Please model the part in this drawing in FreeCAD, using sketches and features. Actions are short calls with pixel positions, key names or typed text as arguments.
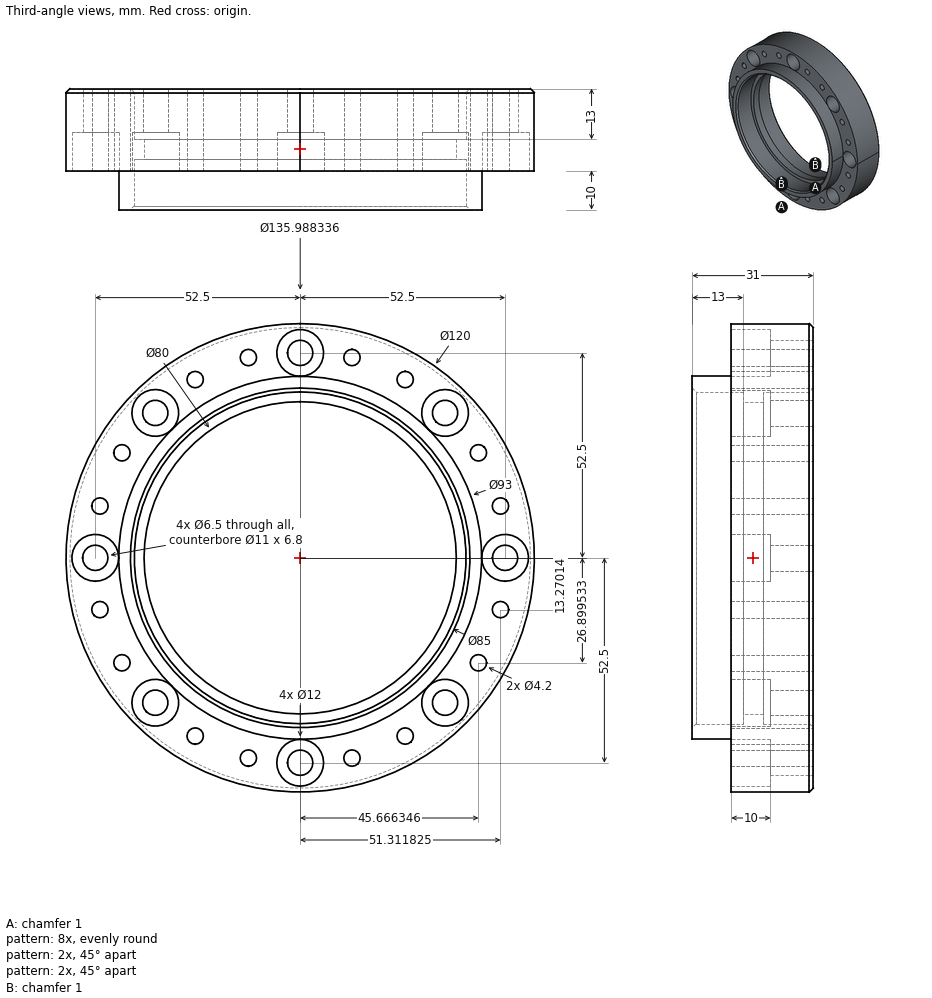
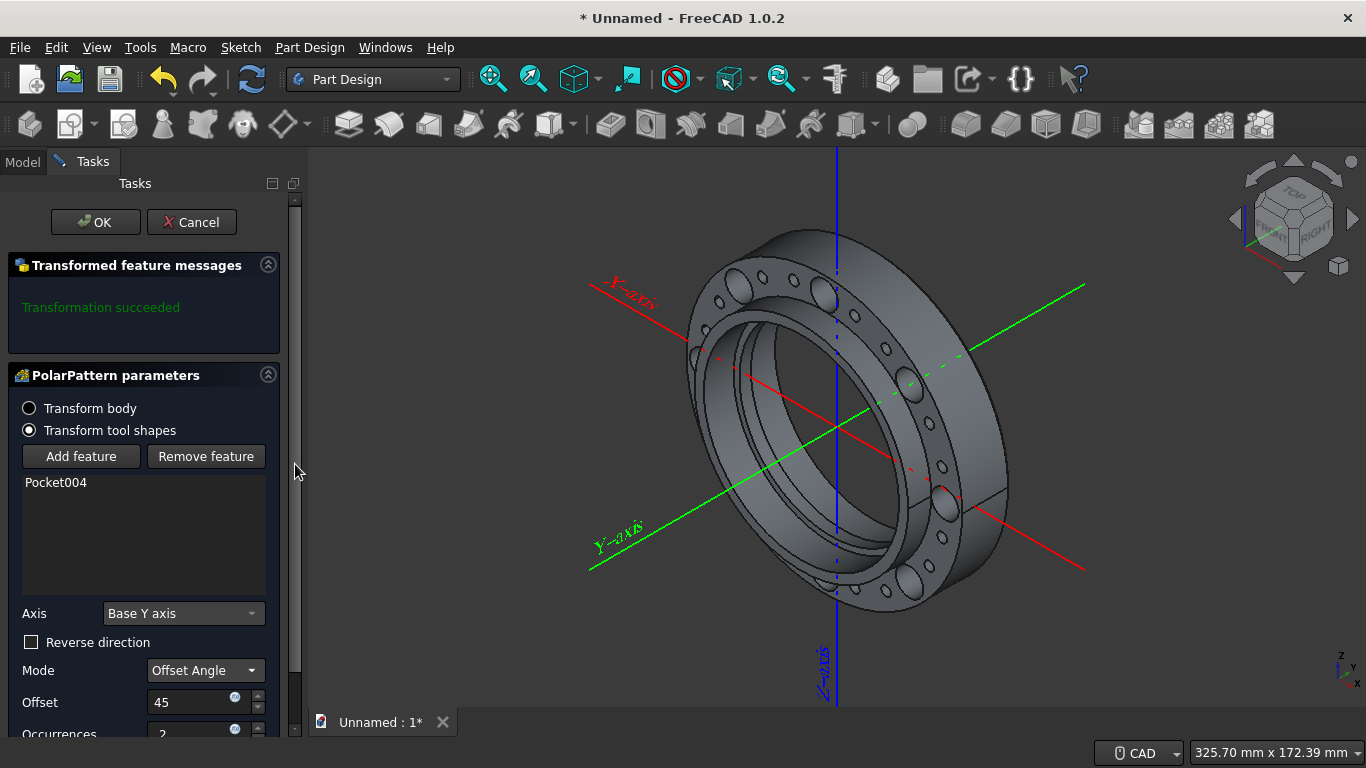
click(96, 222)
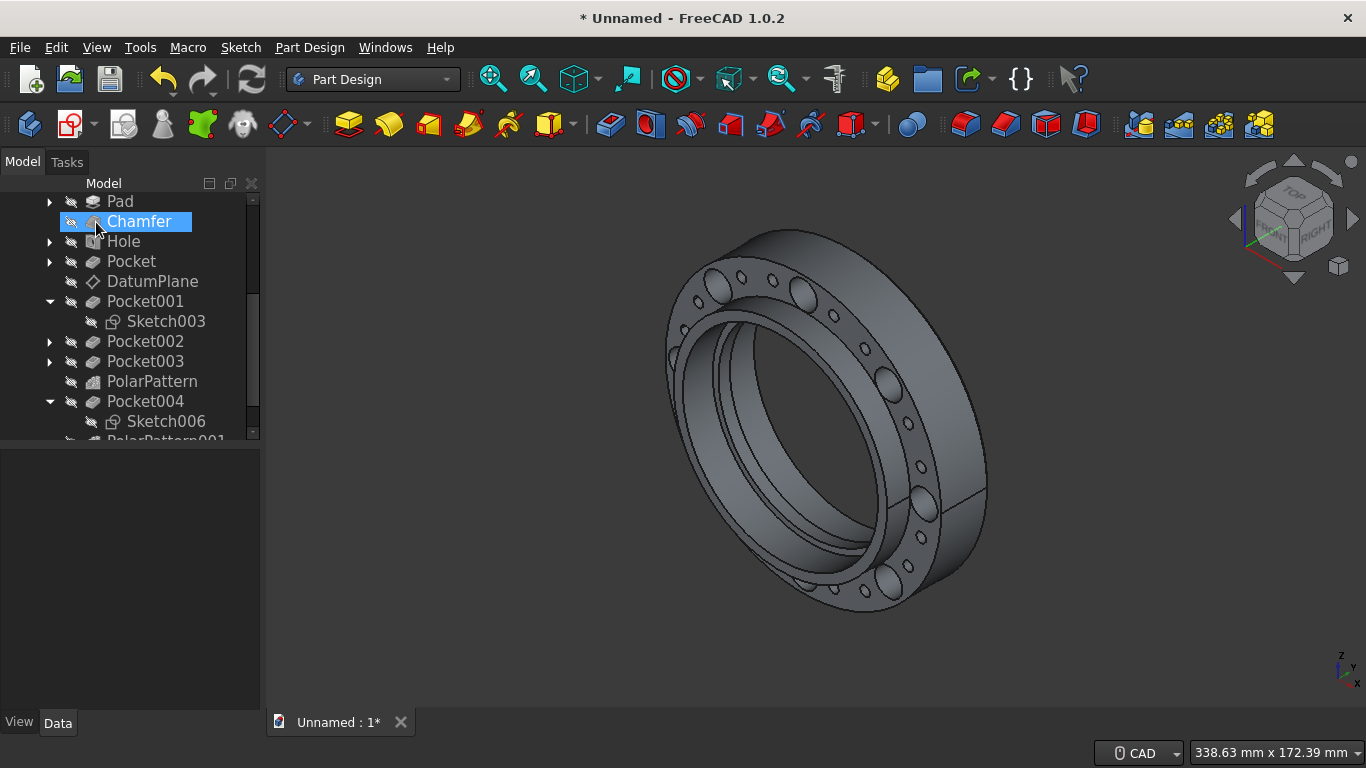
click(683, 390)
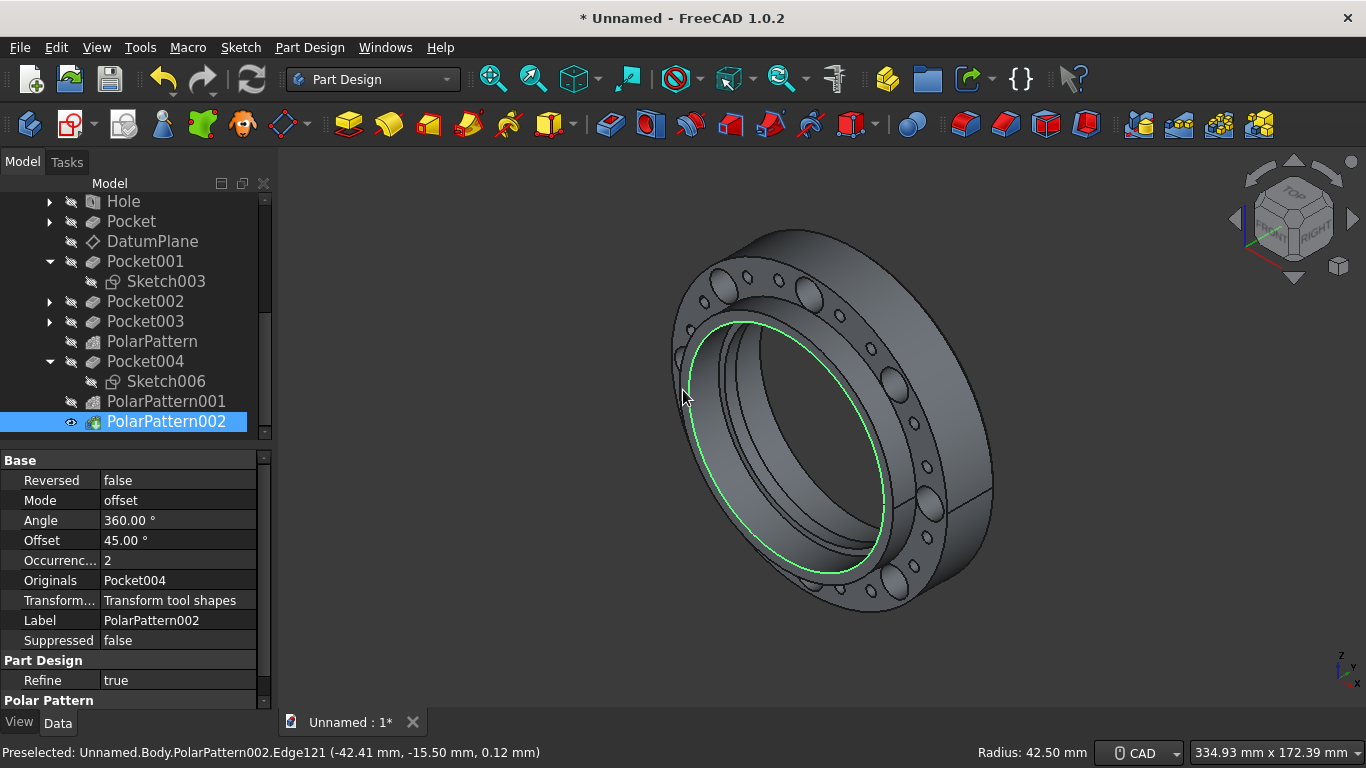
key(2)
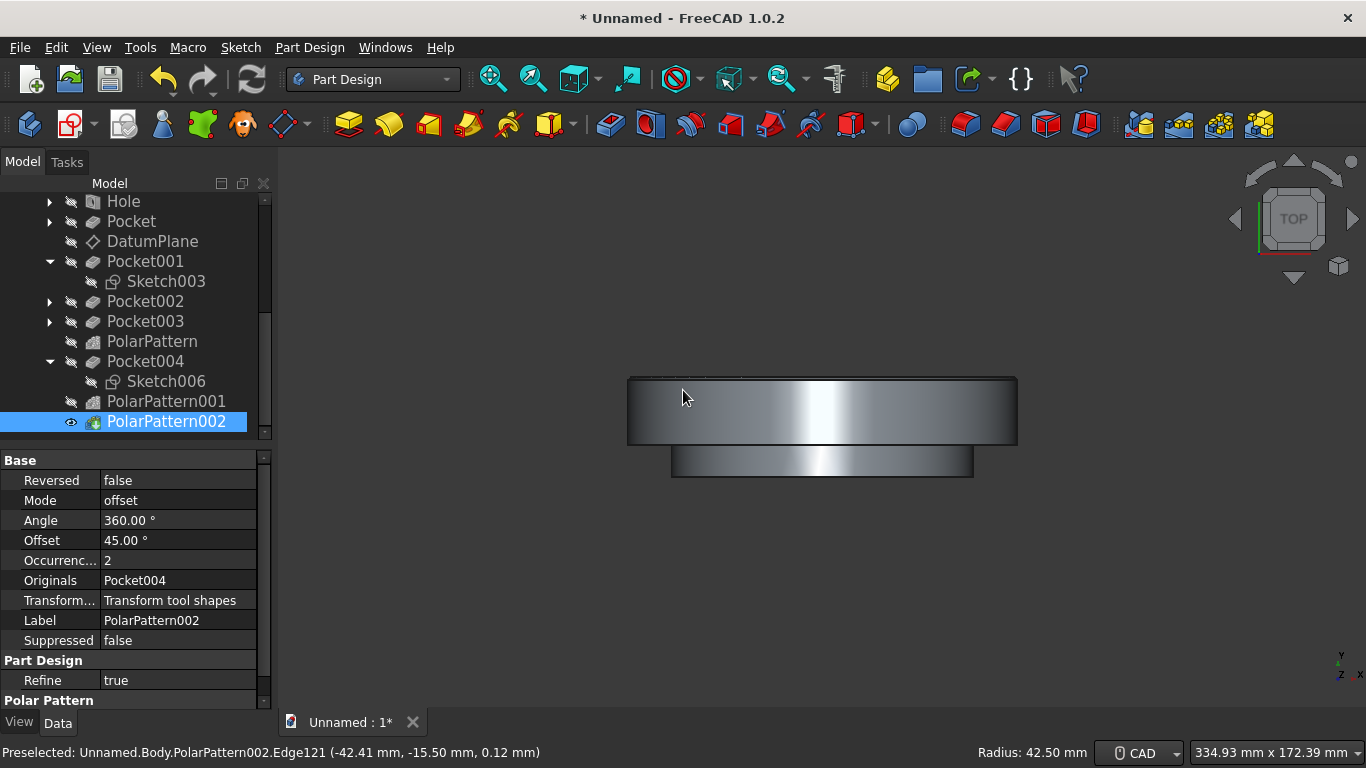
click(494, 80)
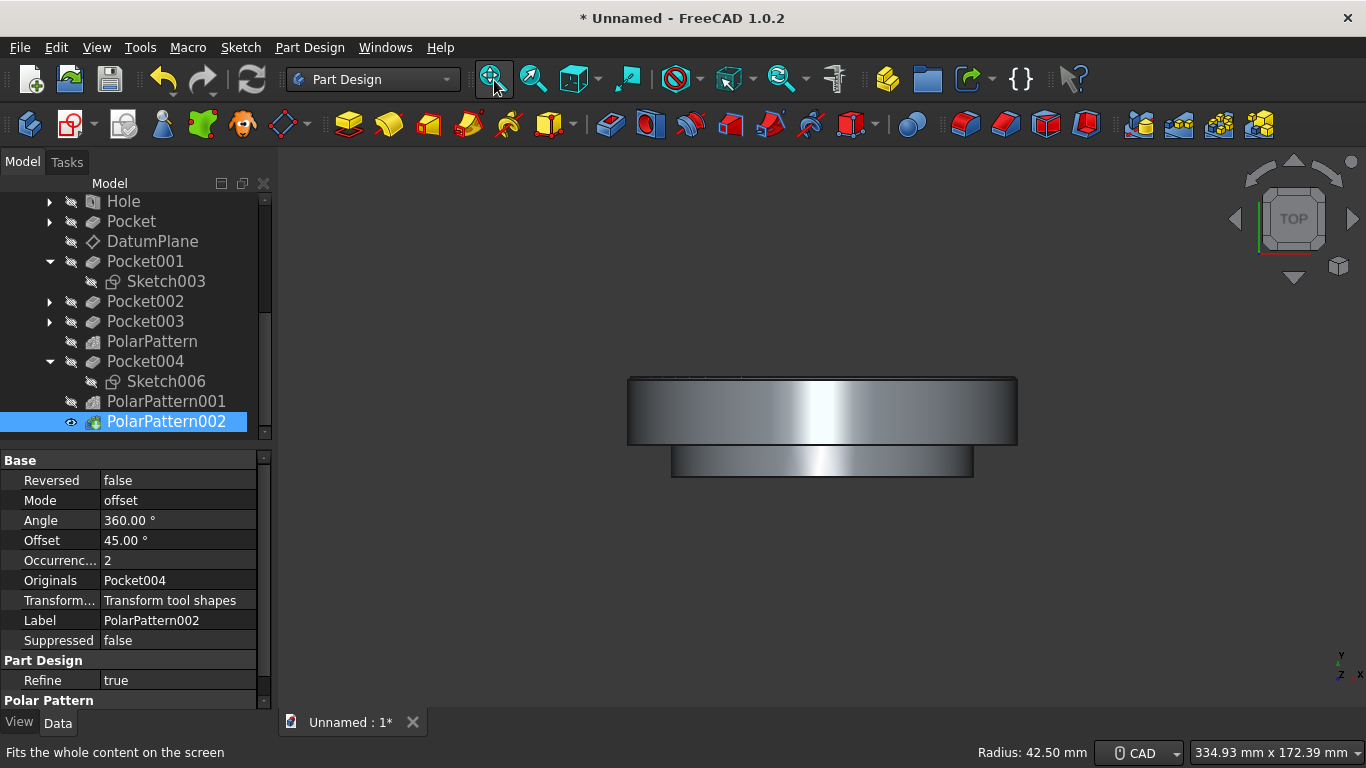
key(0)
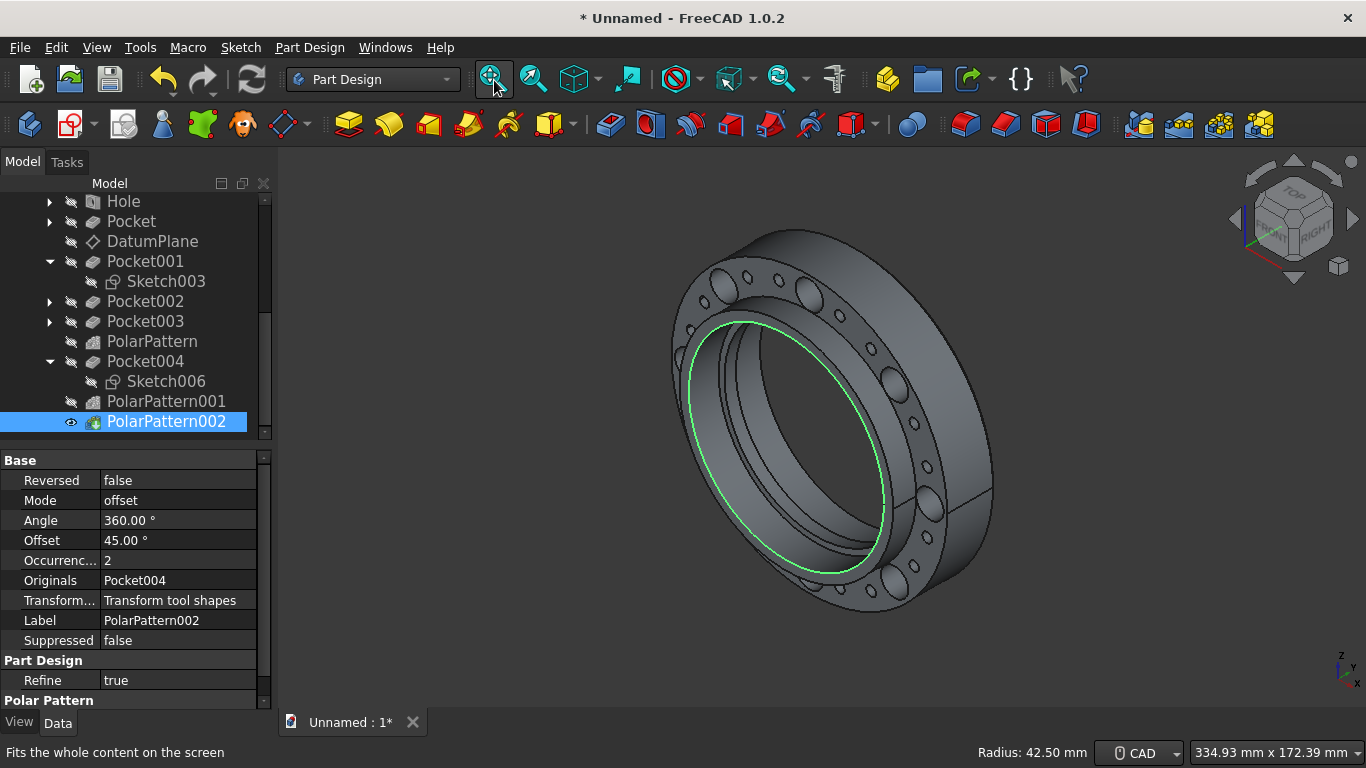
key(1)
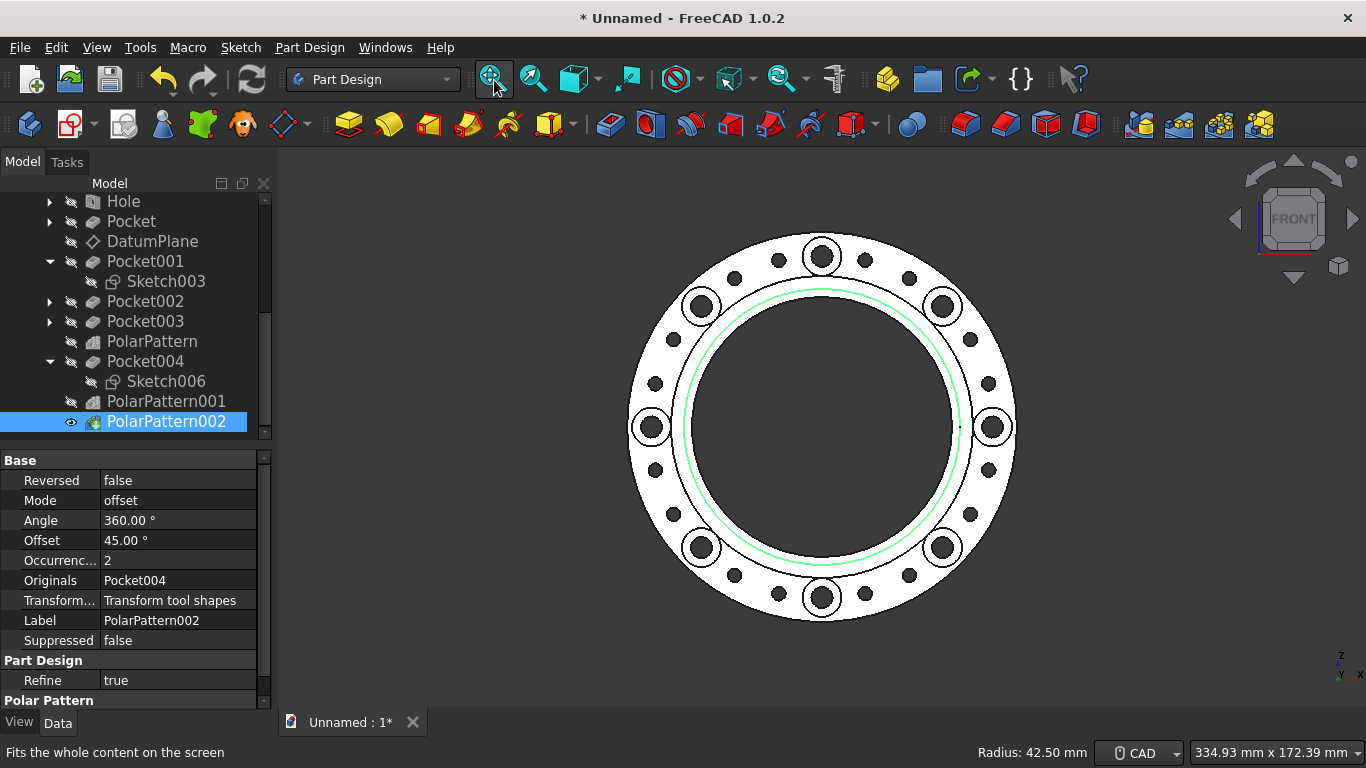
key(3)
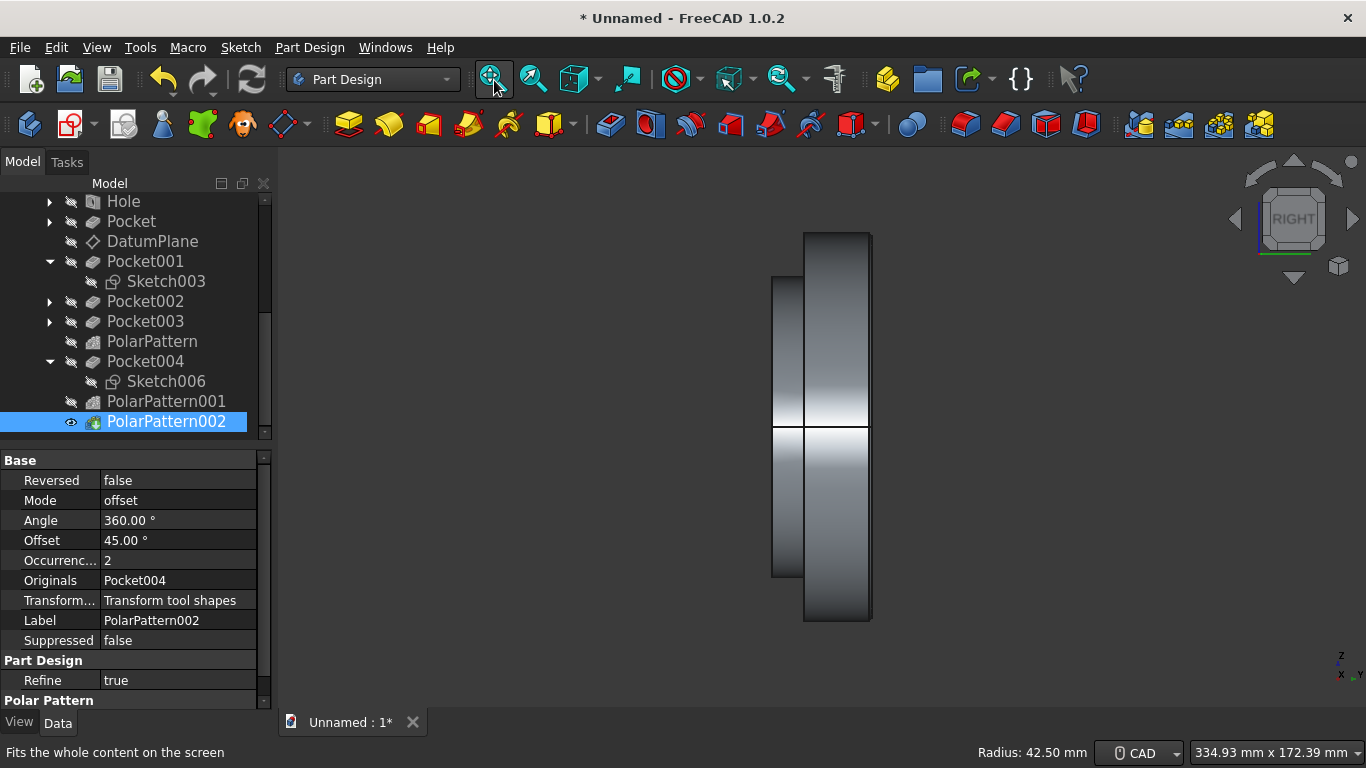
key(5)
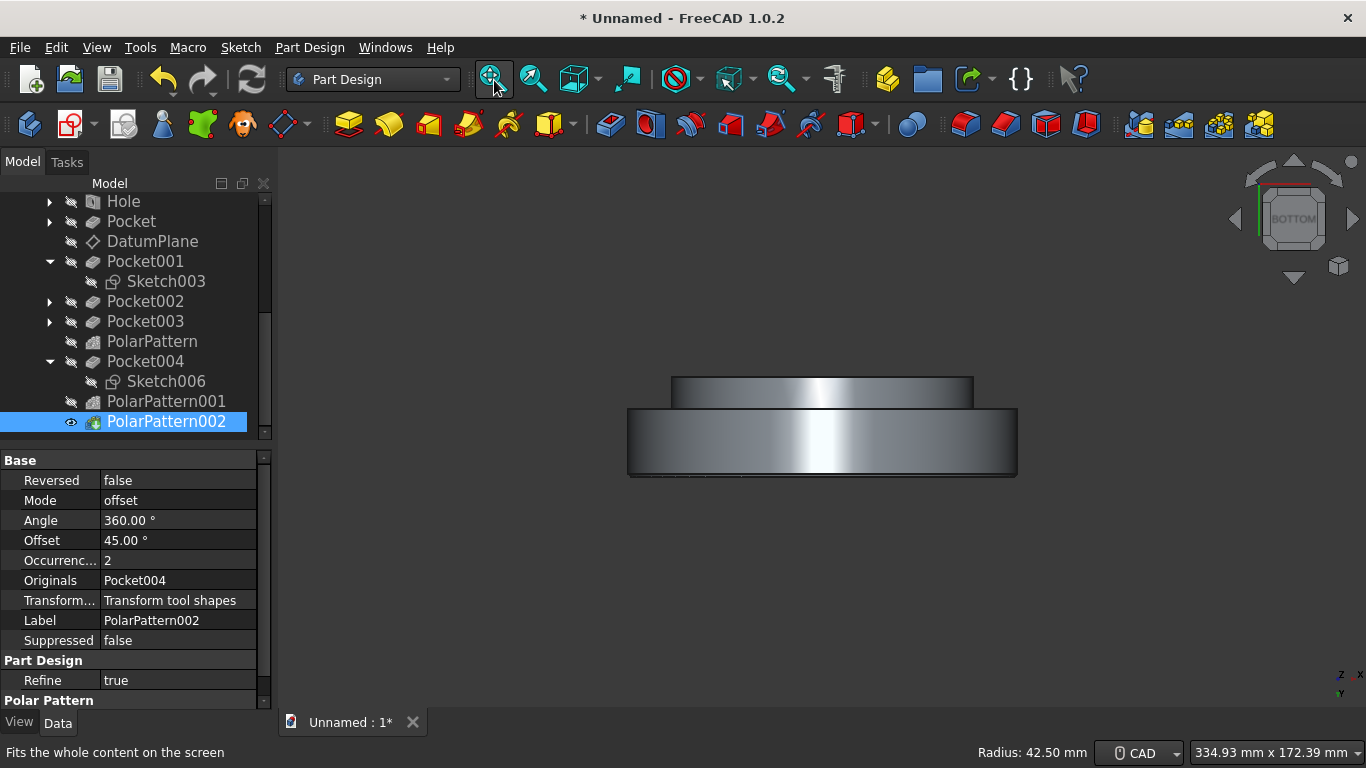
click(494, 80)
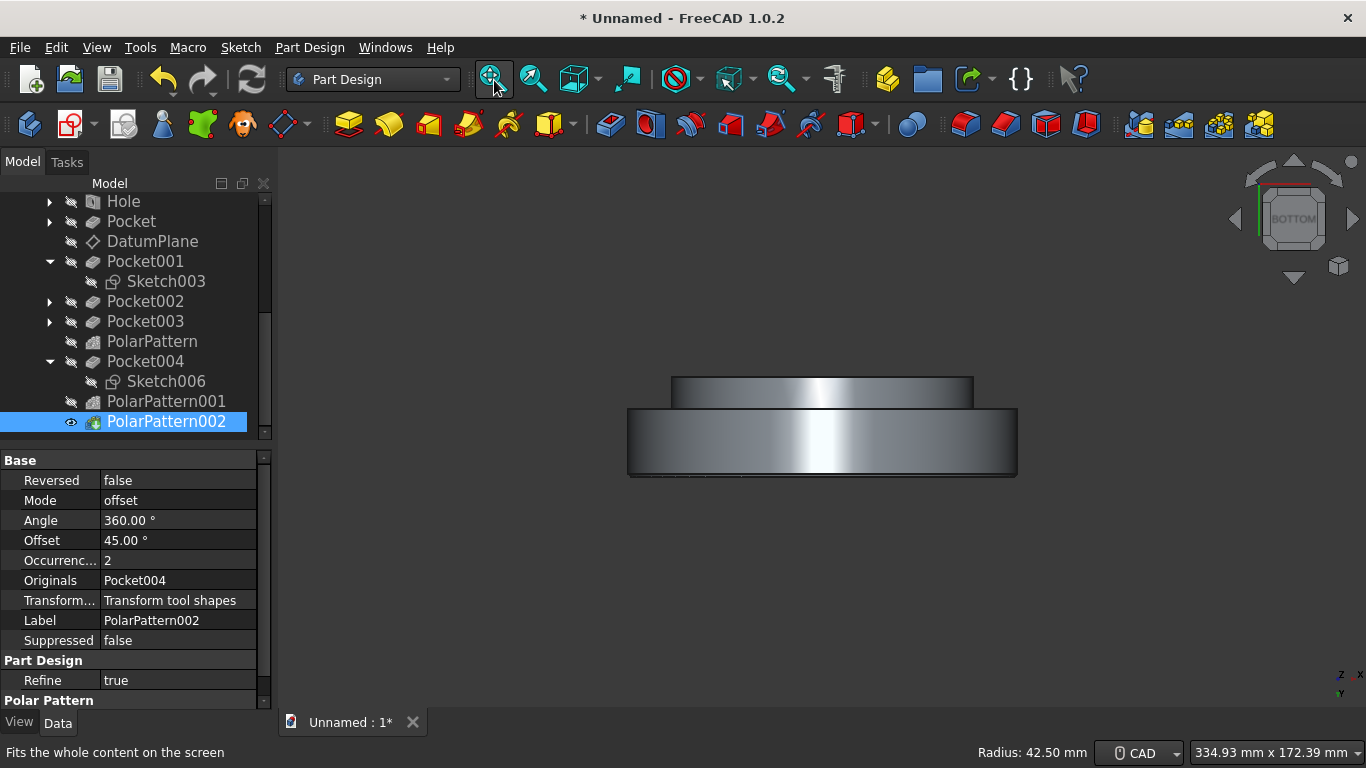
key(4)